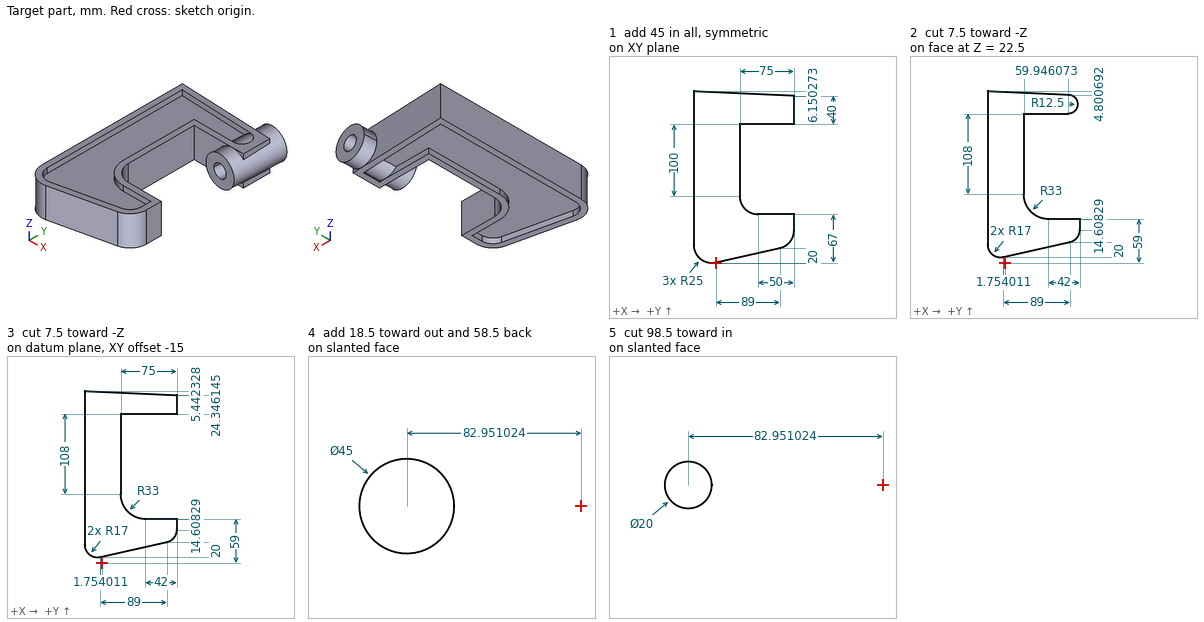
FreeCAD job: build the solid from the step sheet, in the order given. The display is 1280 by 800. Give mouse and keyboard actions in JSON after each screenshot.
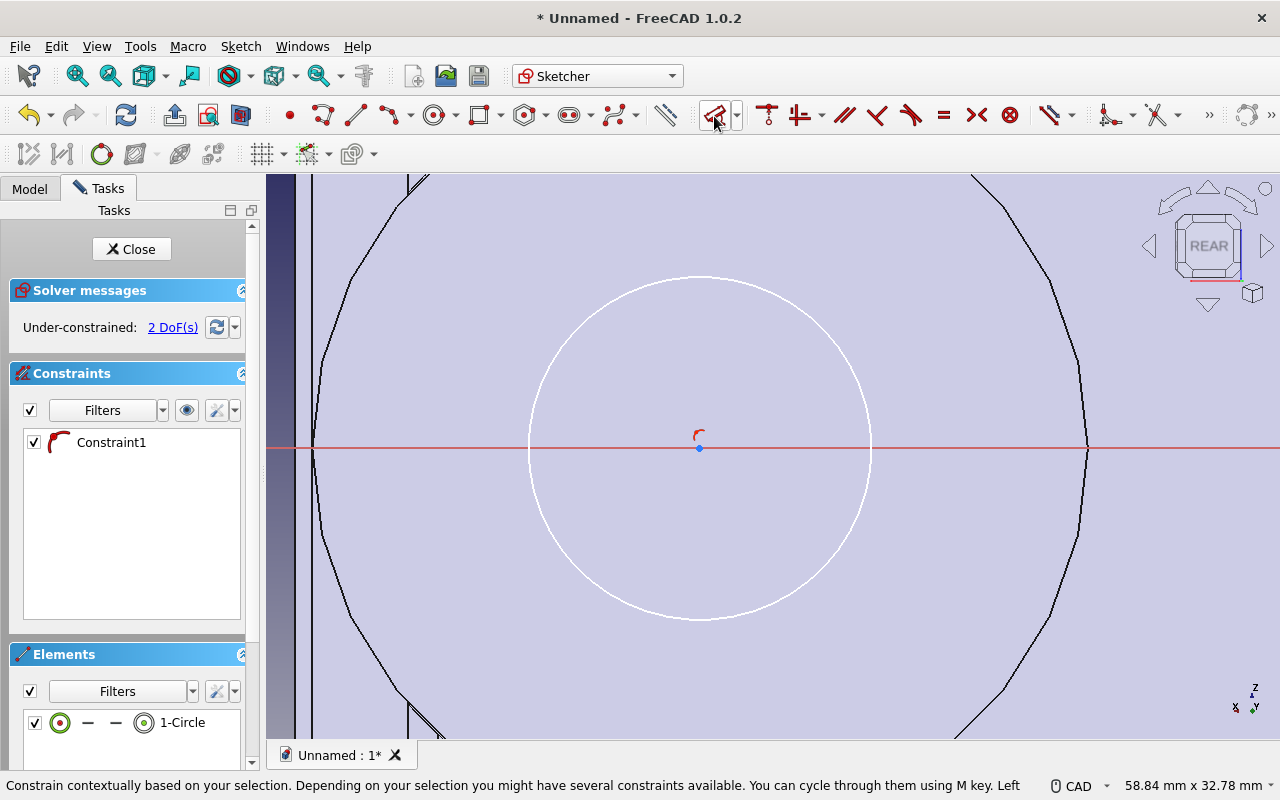
{"action": "left_click", "coordinate": [821, 327]}
{"action": "left_click", "coordinate": [844, 304]}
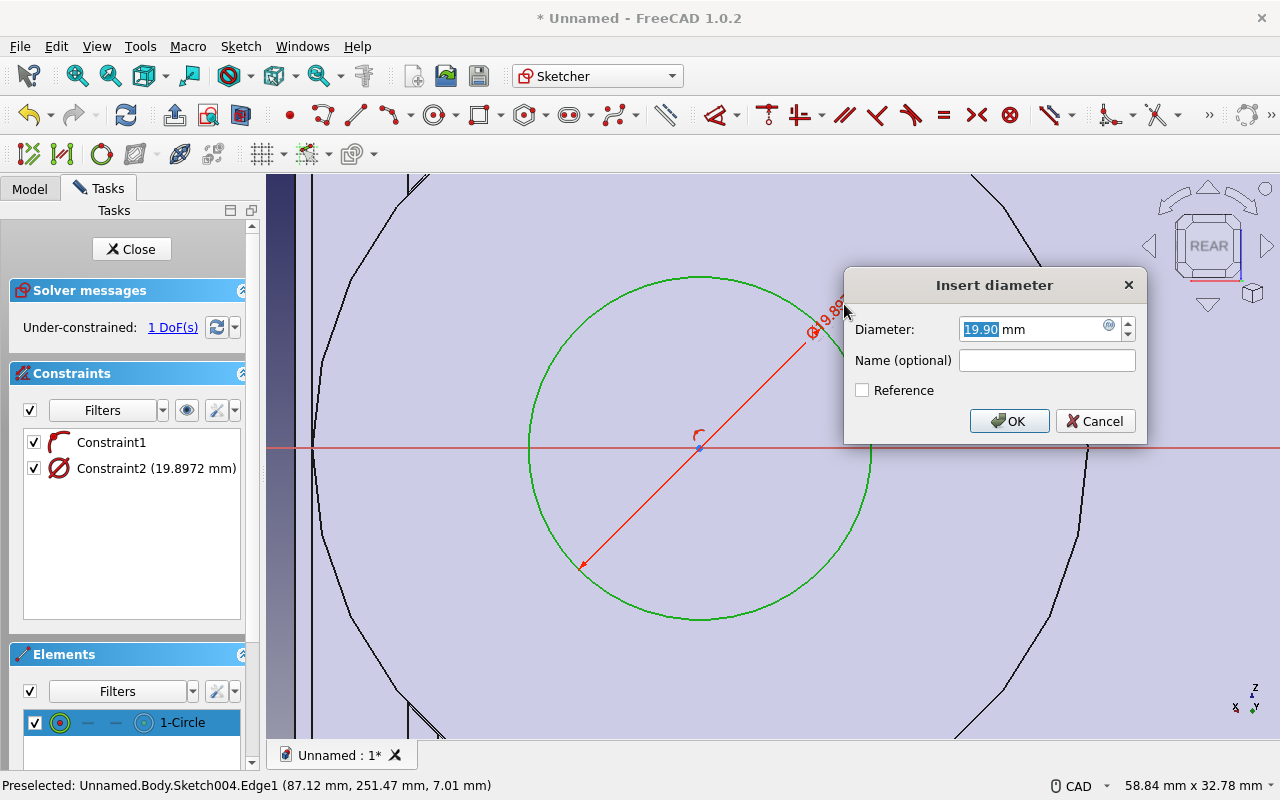
{"action": "type", "text": "20"}
{"action": "key", "text": "Return"}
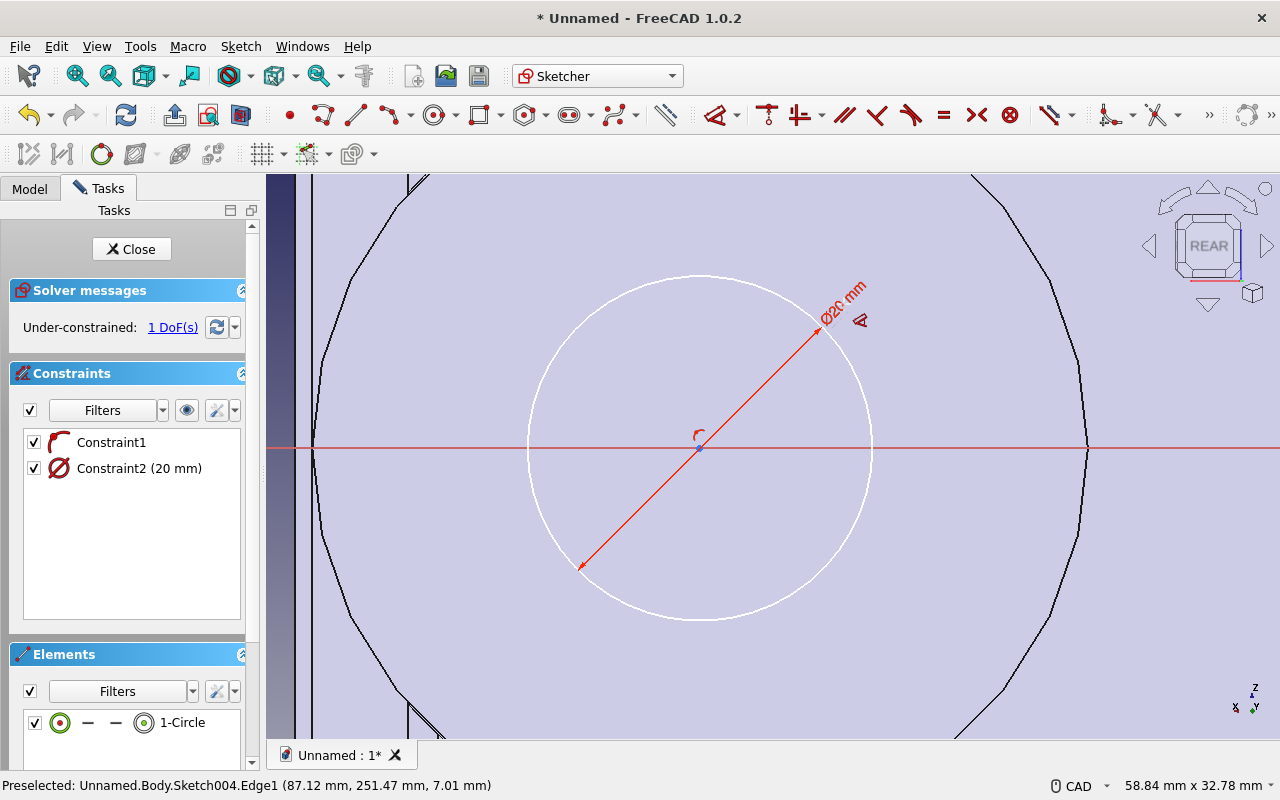
{"action": "left_click", "coordinate": [700, 448]}
{"action": "left_click", "coordinate": [907, 482]}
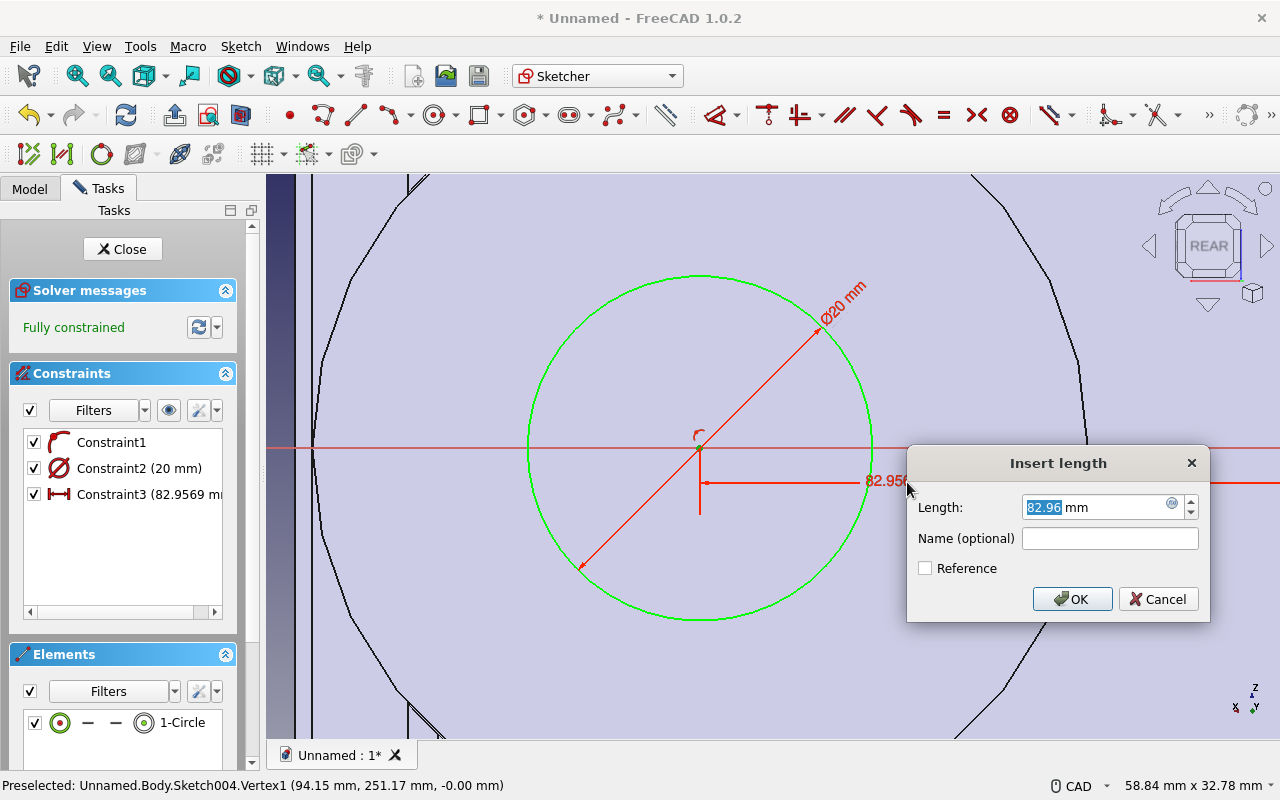
{"action": "type", "text": "82.951024"}
{"action": "key", "text": "Return"}
{"action": "key", "text": "Escape"}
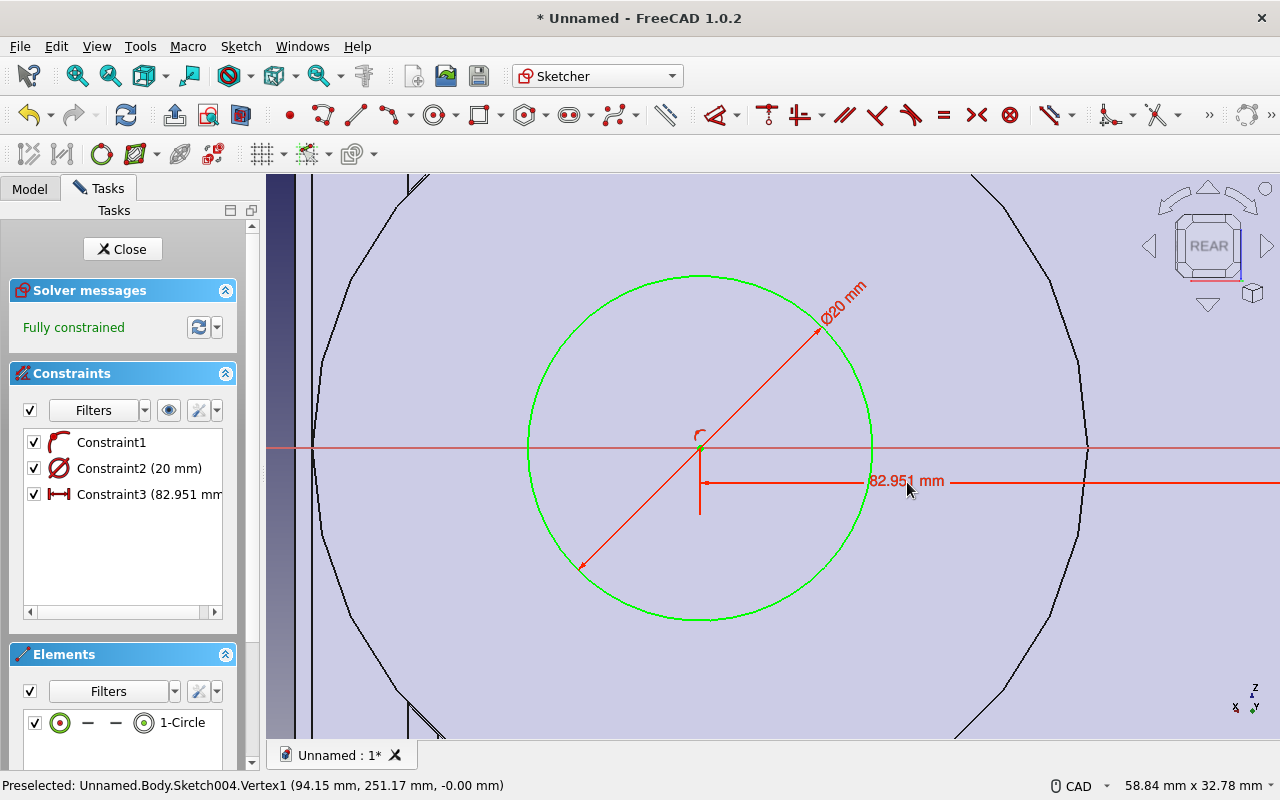
{"action": "left_click", "coordinate": [123, 249]}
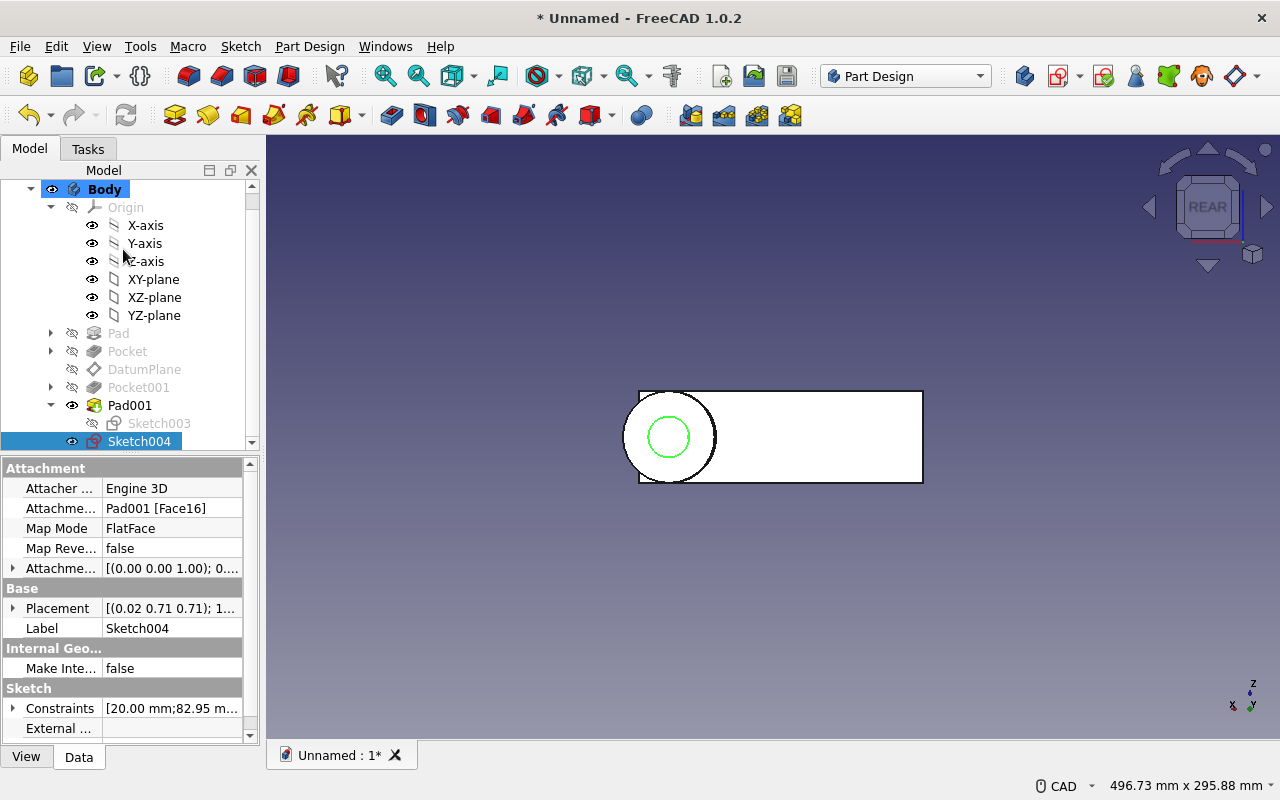
{"action": "left_click", "coordinate": [392, 116]}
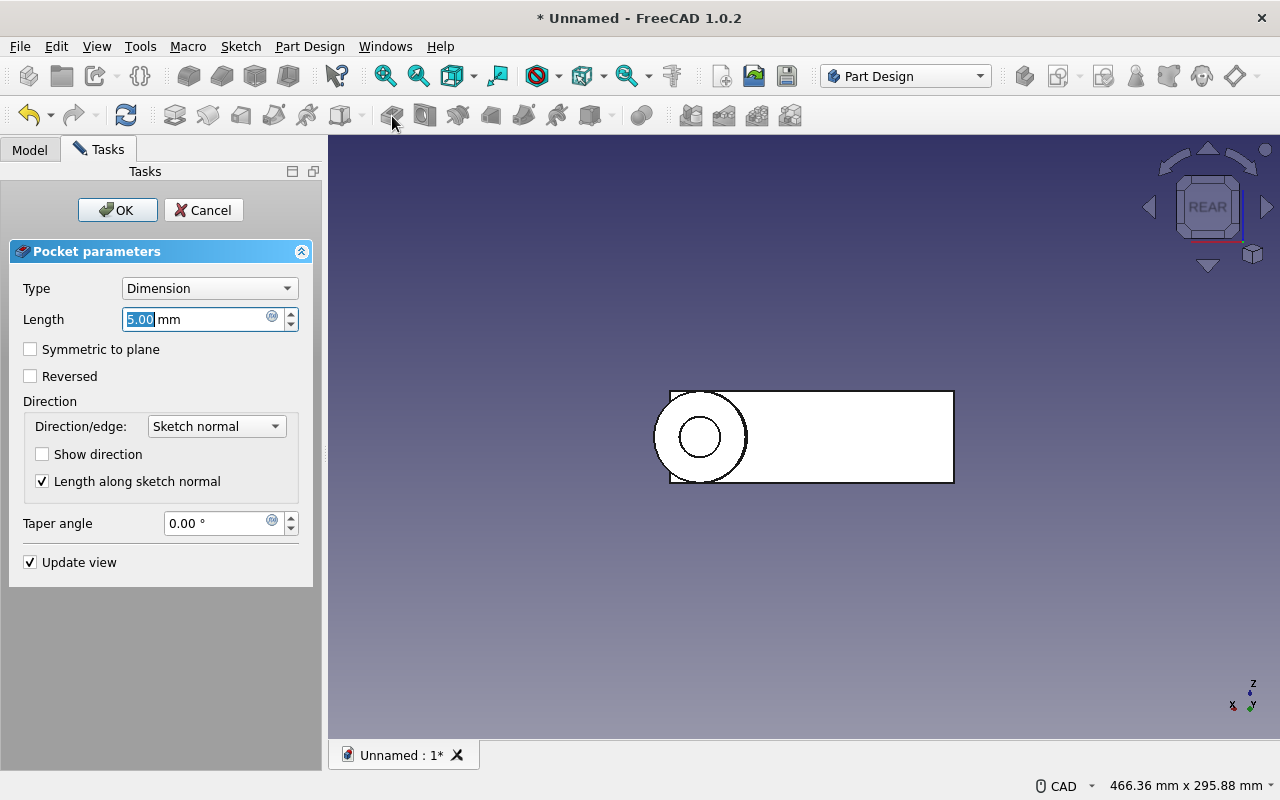
{"action": "type", "text": "98.5"}
{"action": "key", "text": "Tab"}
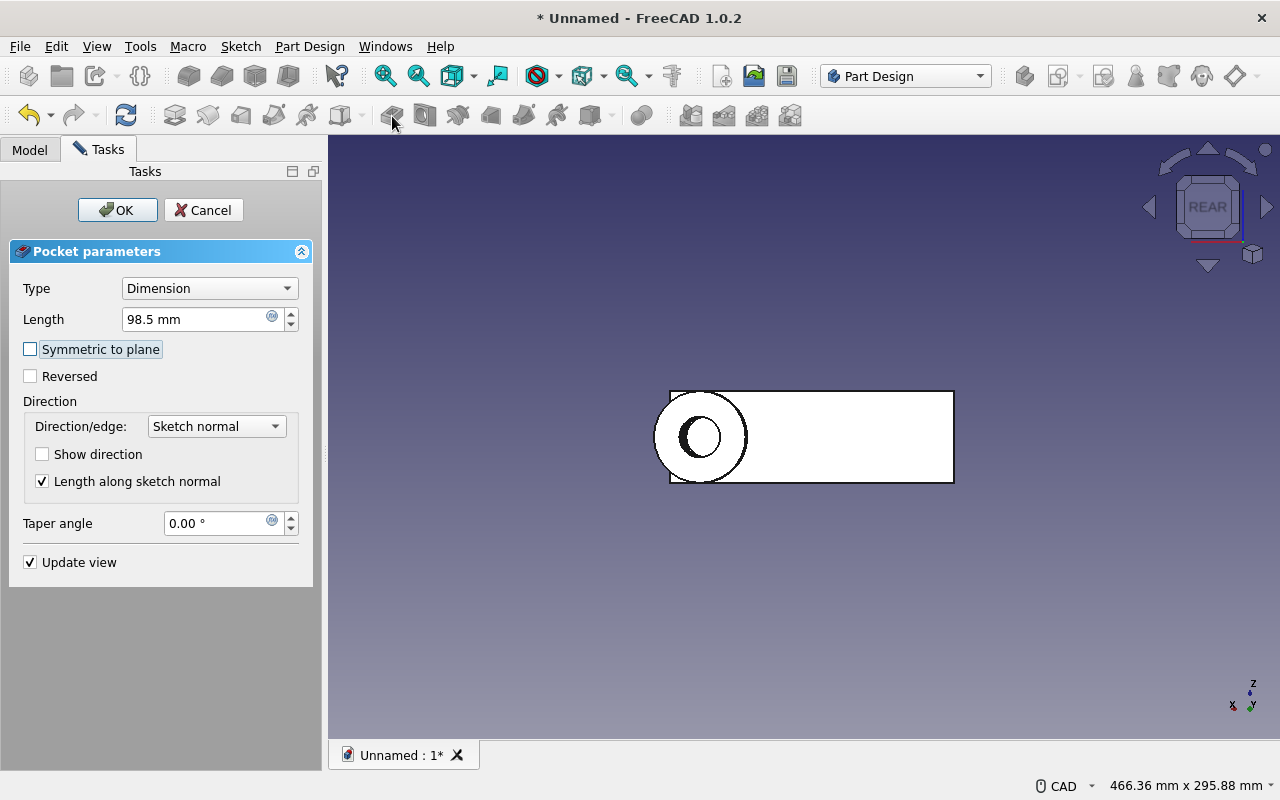
{"action": "left_click", "coordinate": [118, 210]}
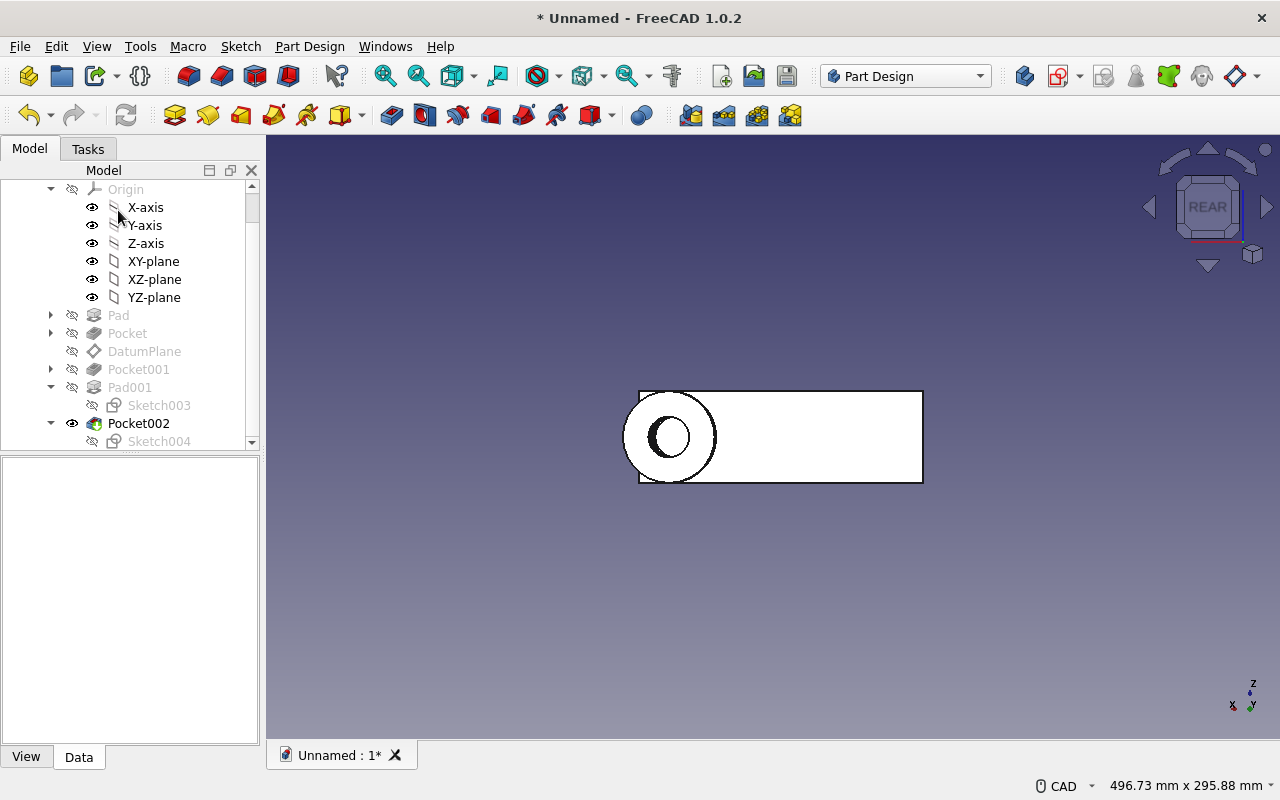
{"action": "key", "text": "0"}